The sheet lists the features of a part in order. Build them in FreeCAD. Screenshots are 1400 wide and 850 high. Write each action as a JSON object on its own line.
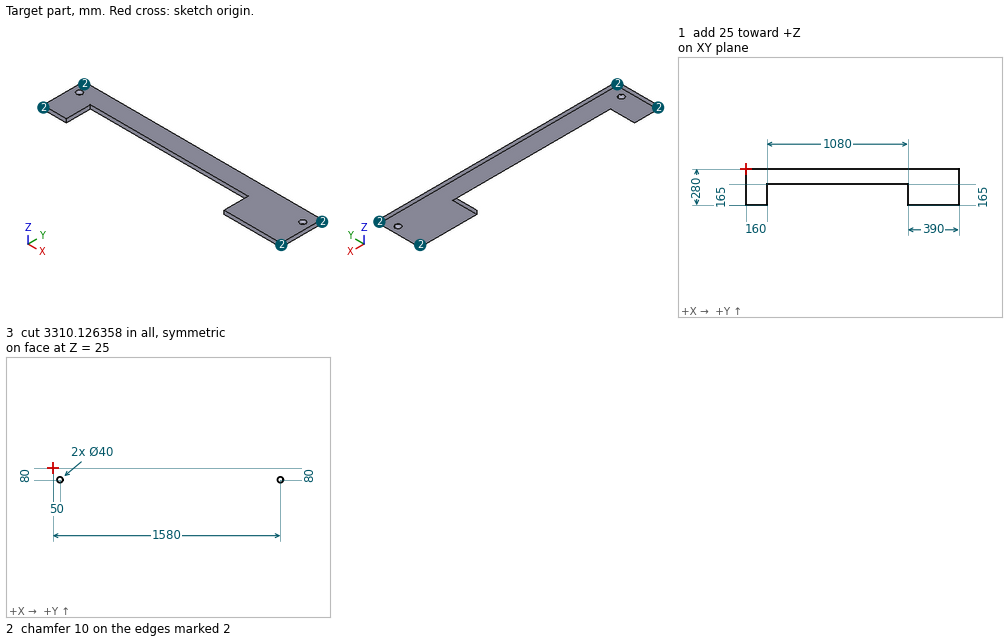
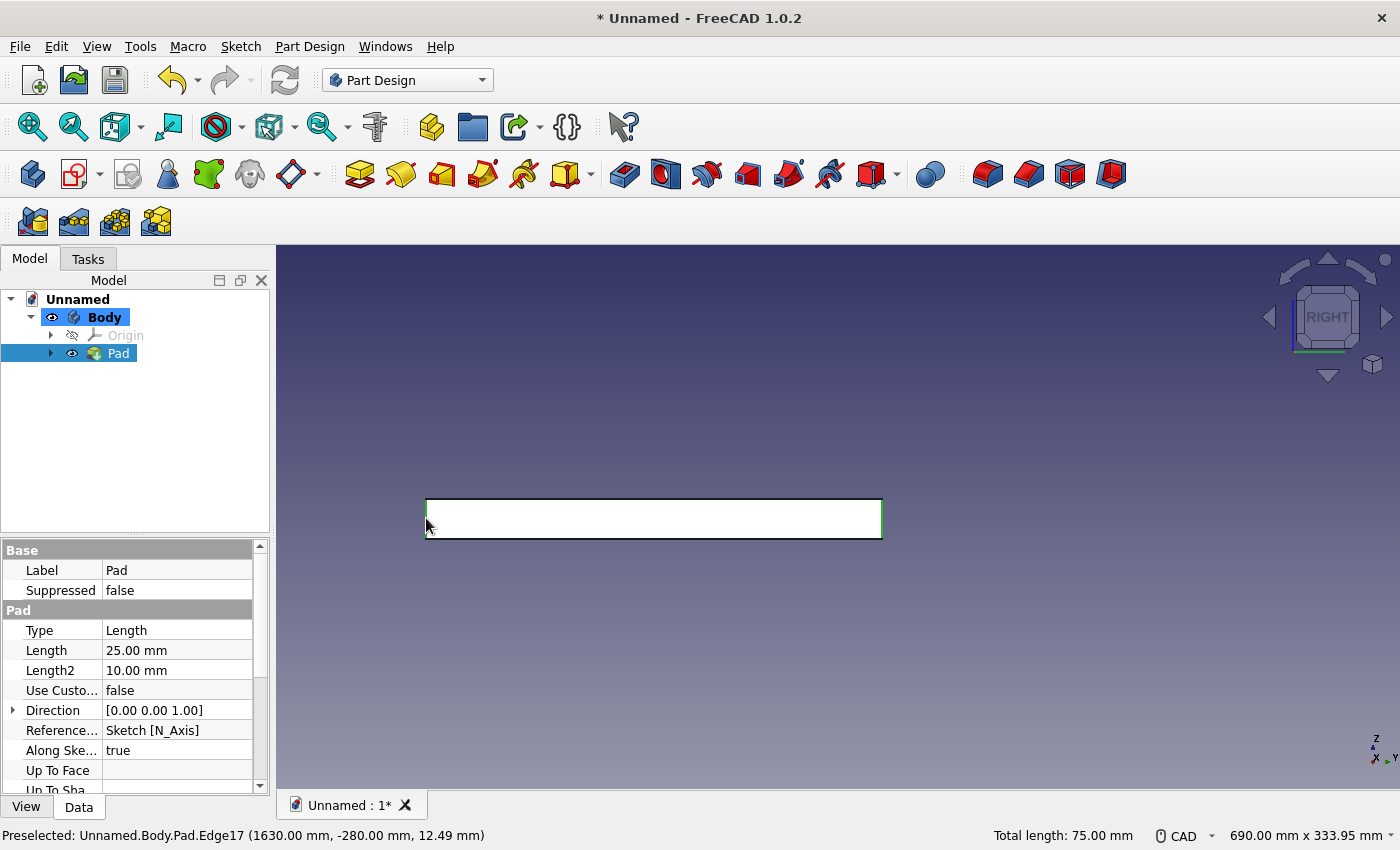
{"action": "key", "text": "v f"}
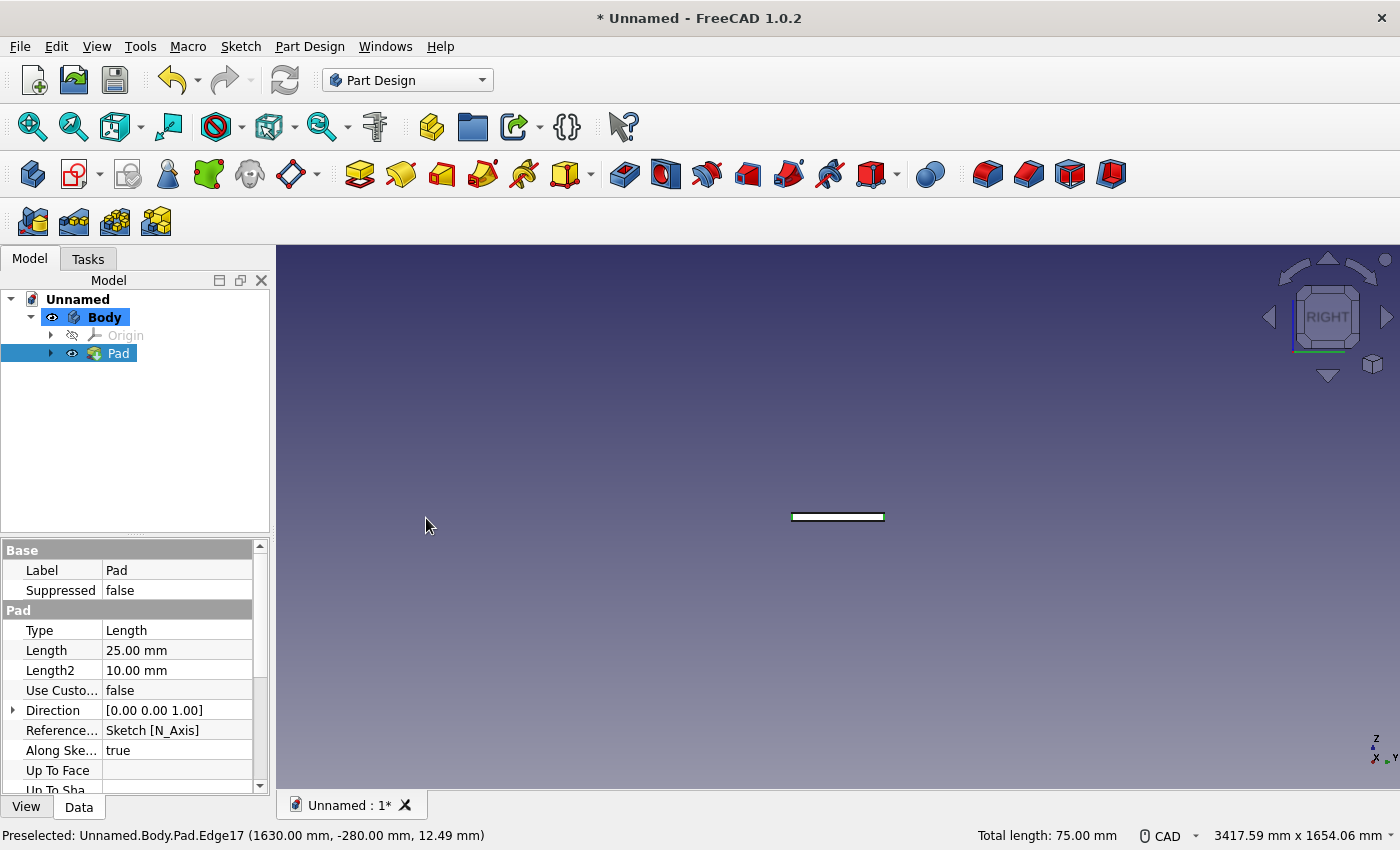
{"action": "key", "text": "5"}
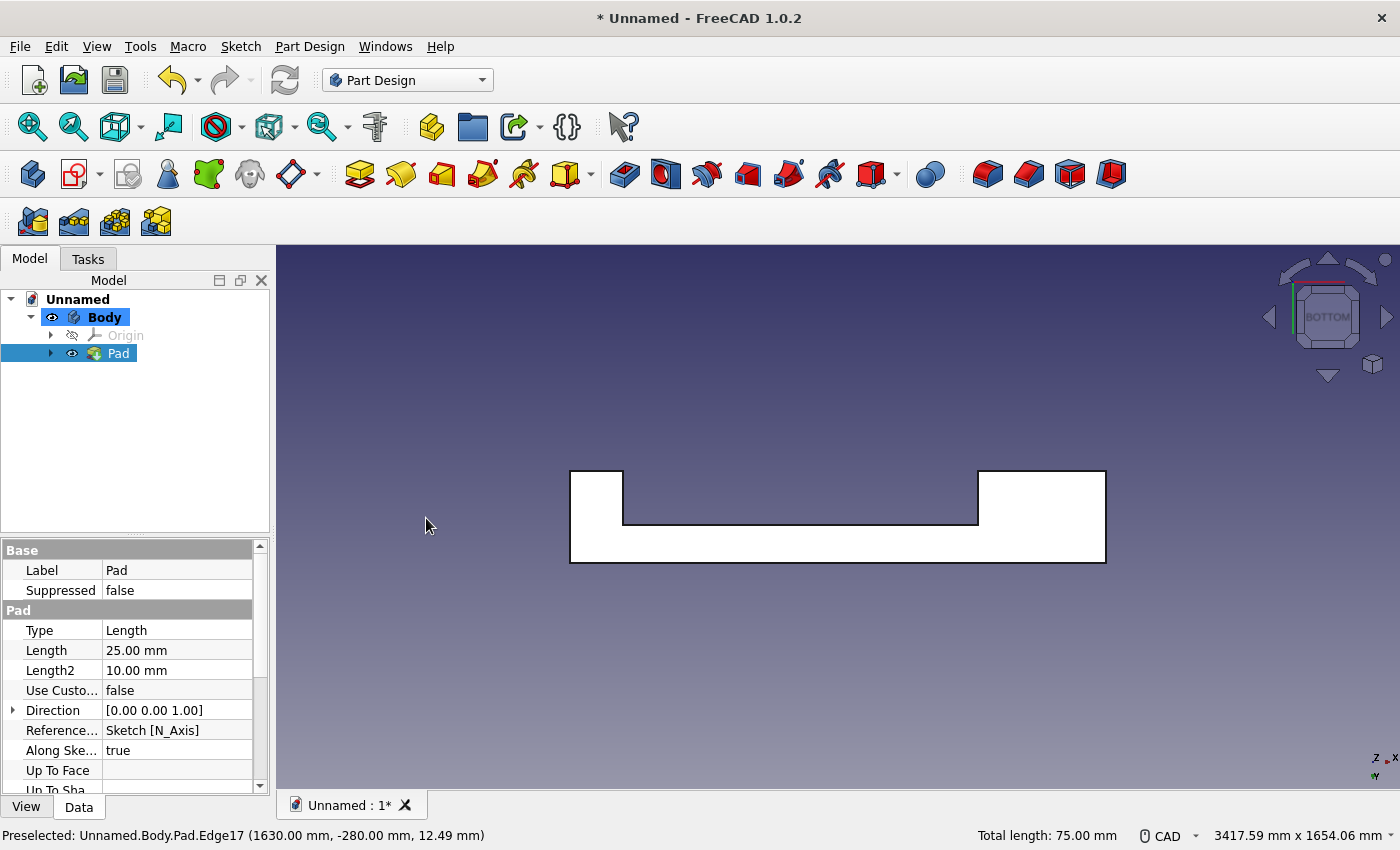
{"action": "scroll", "coordinate": [570, 562], "scroll_direction": "up", "scroll_amount": 8}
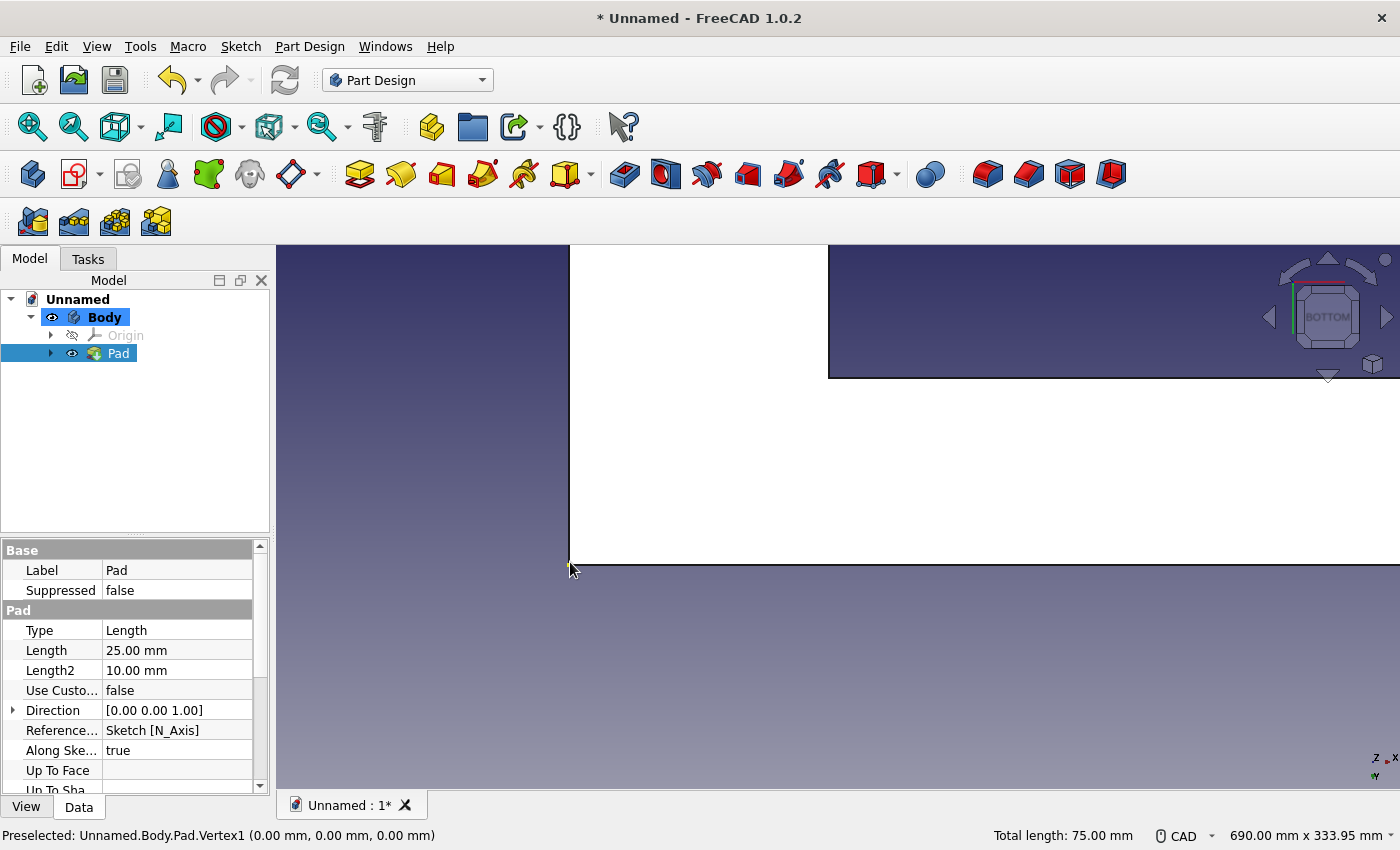
{"action": "key", "text": "v f"}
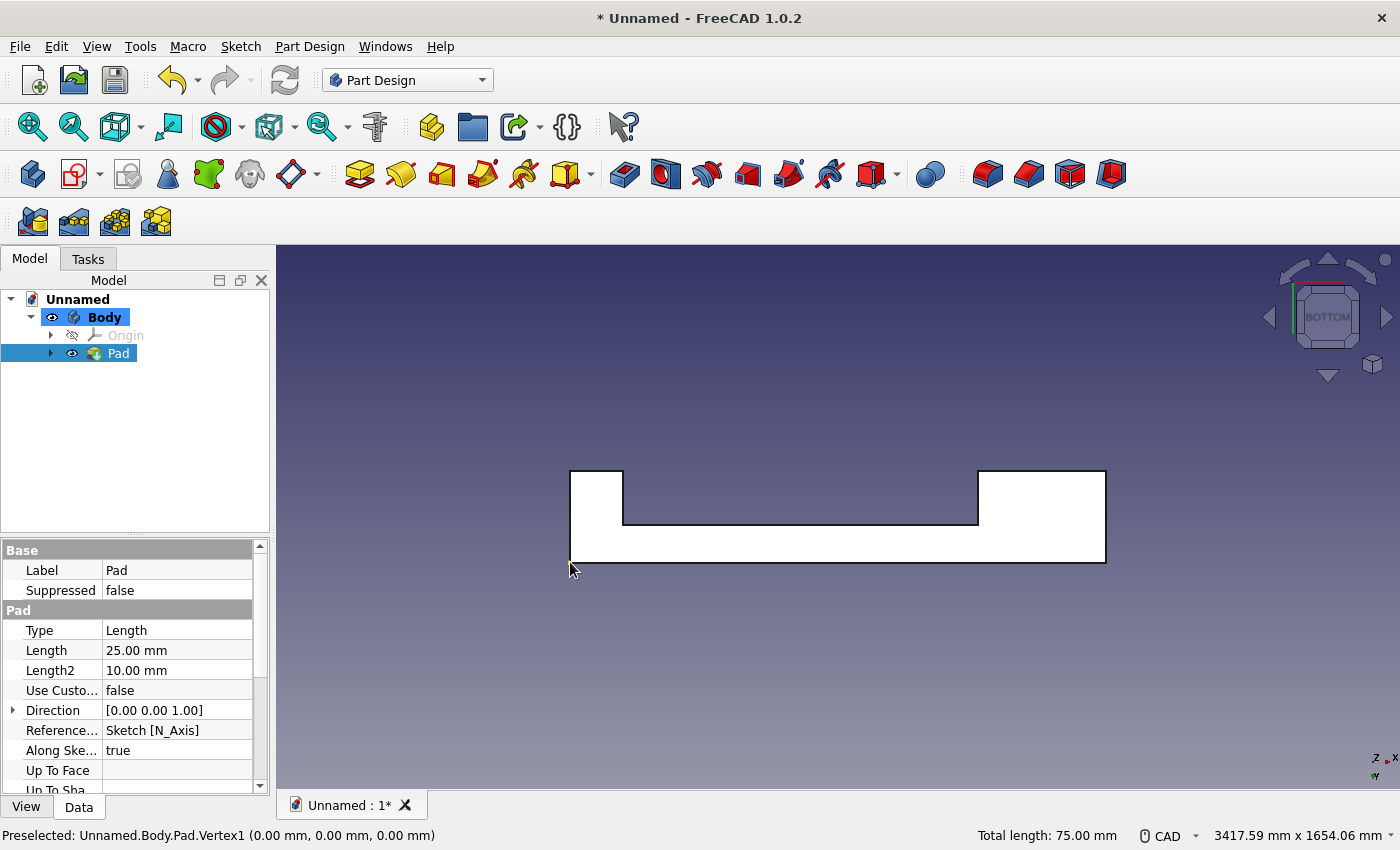
{"action": "key", "text": "4"}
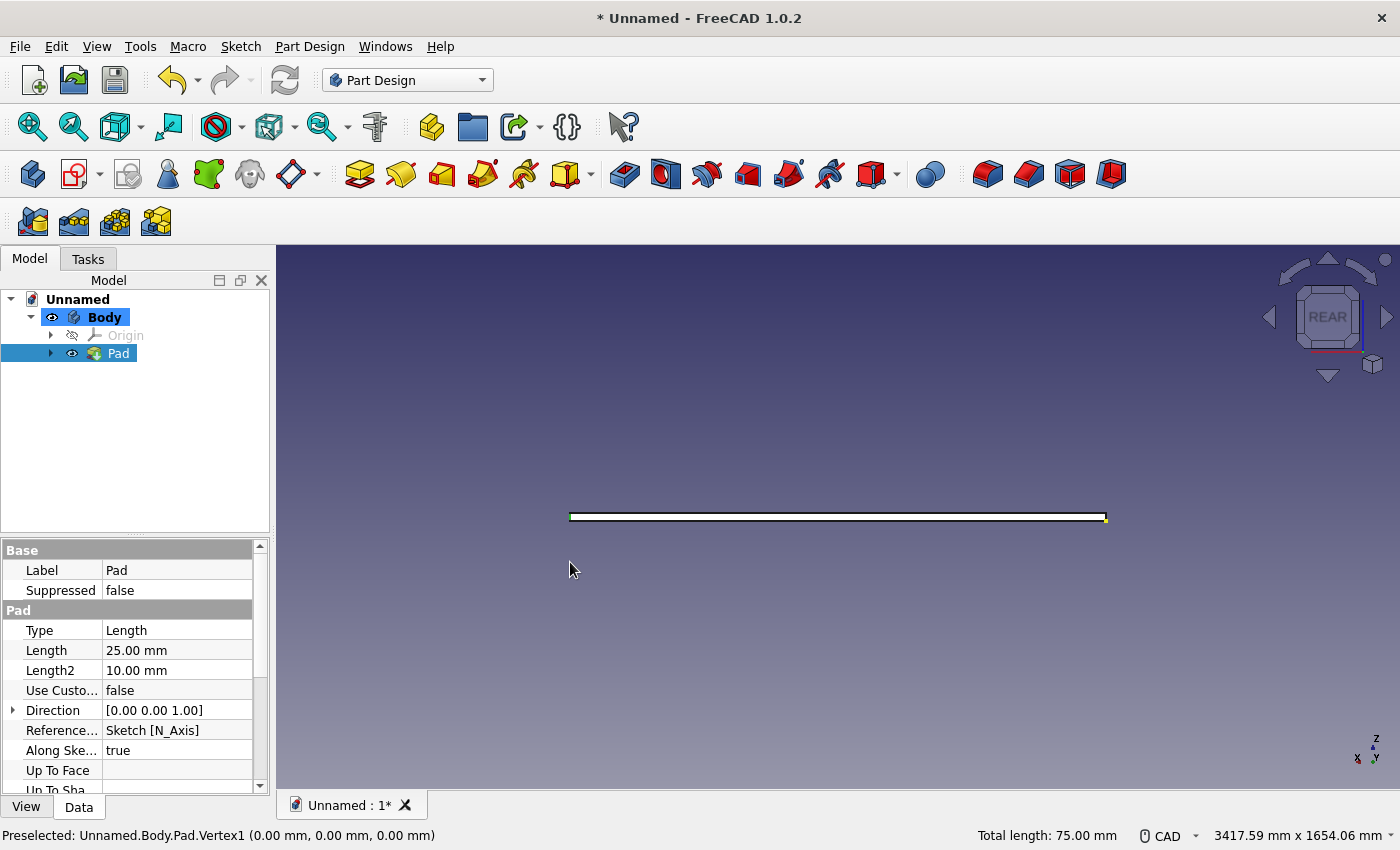
{"action": "scroll", "coordinate": [1106, 516], "scroll_direction": "up", "scroll_amount": 8}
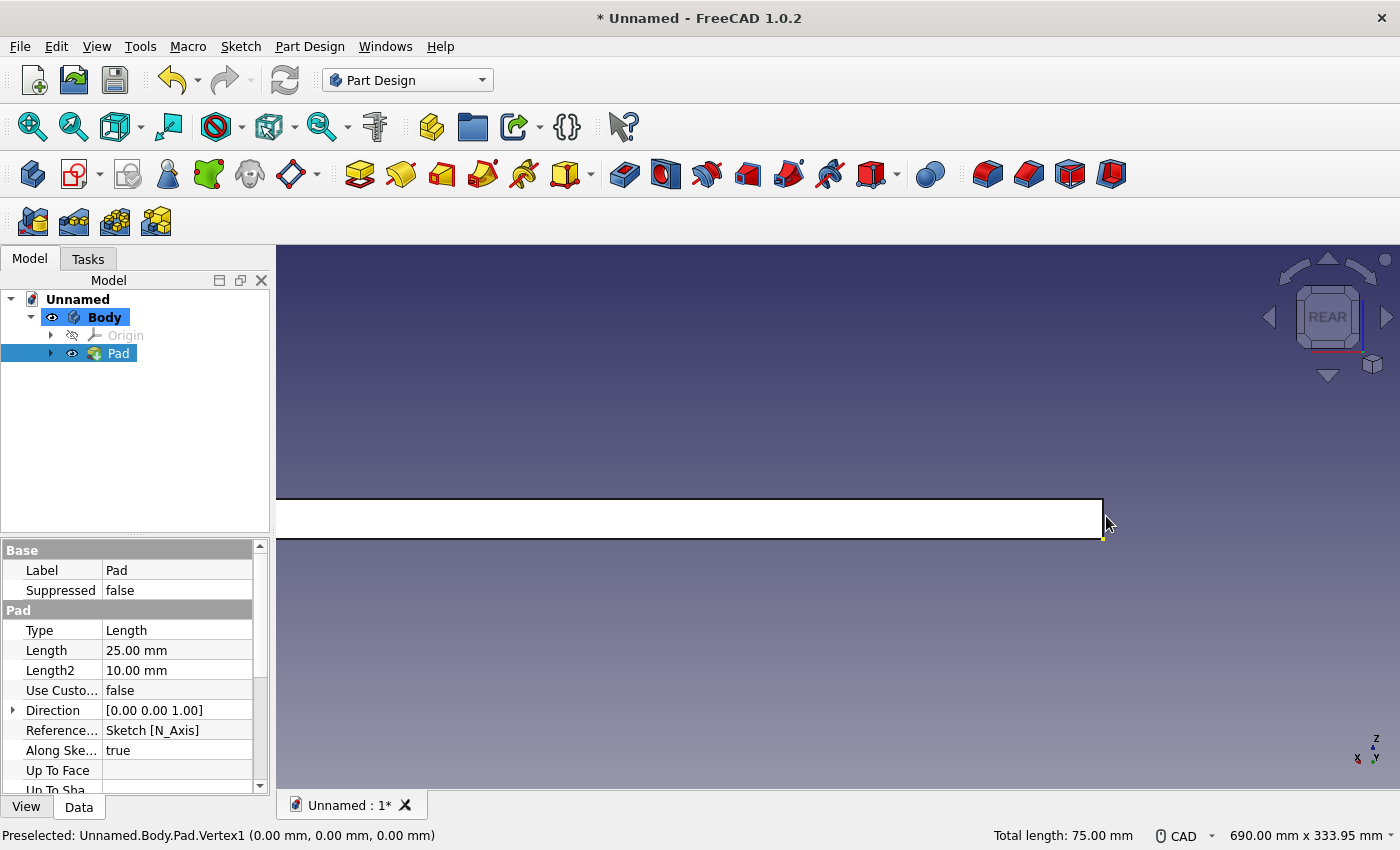
{"action": "left_click", "coordinate": [1103, 518], "text": "ctrl"}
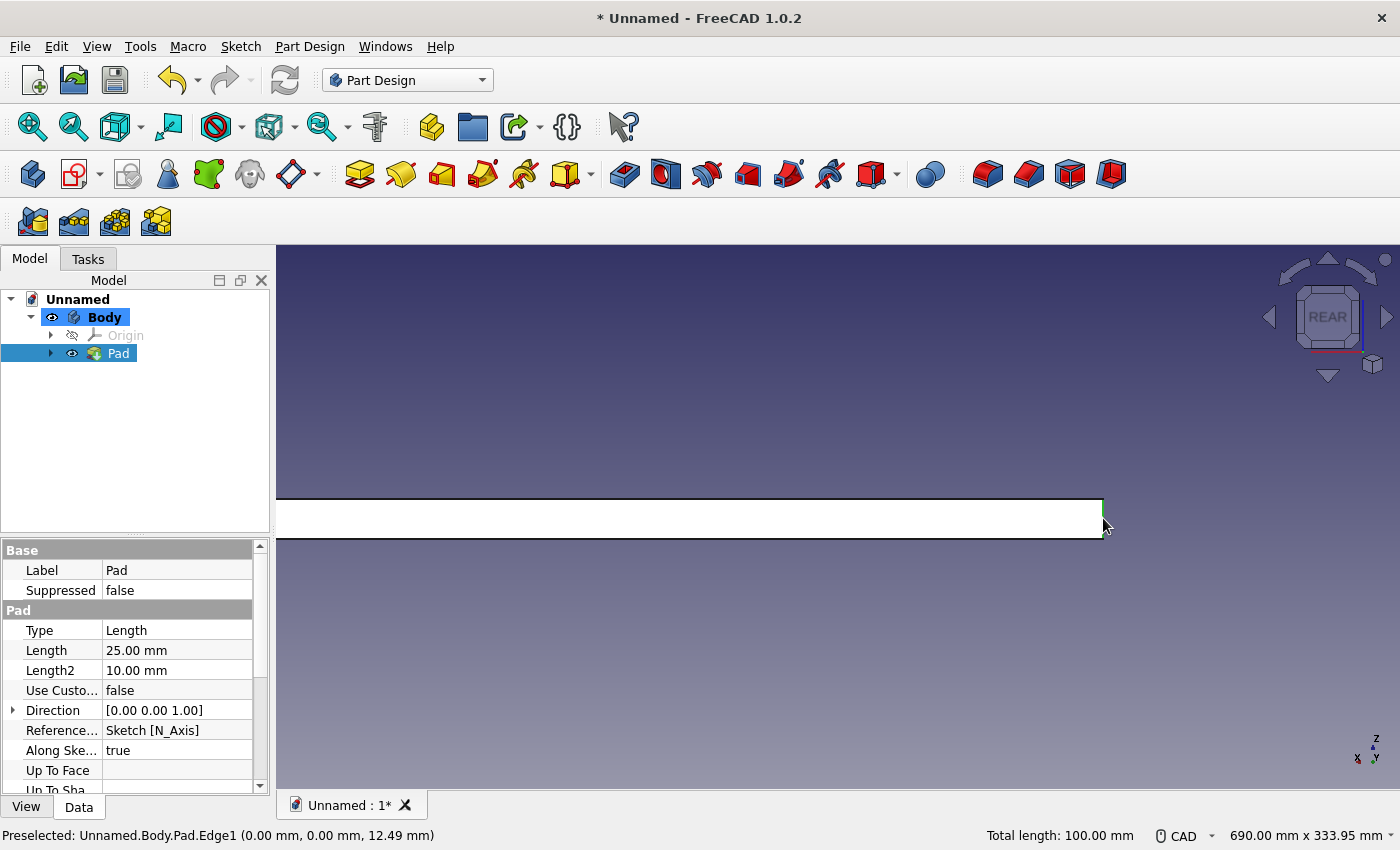
{"action": "left_click", "coordinate": [1029, 174]}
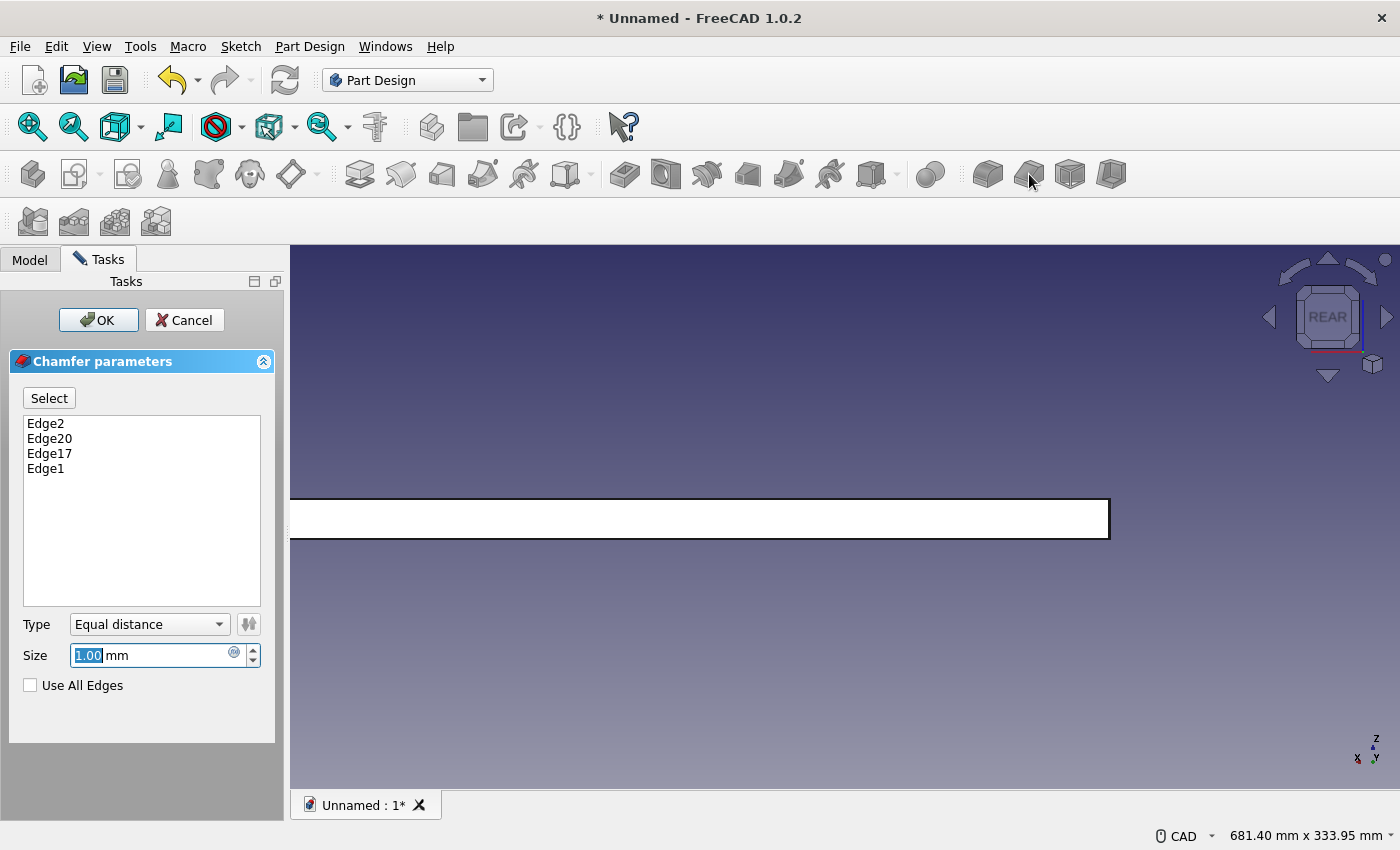
{"action": "type", "text": "10"}
{"action": "key", "text": "Tab"}